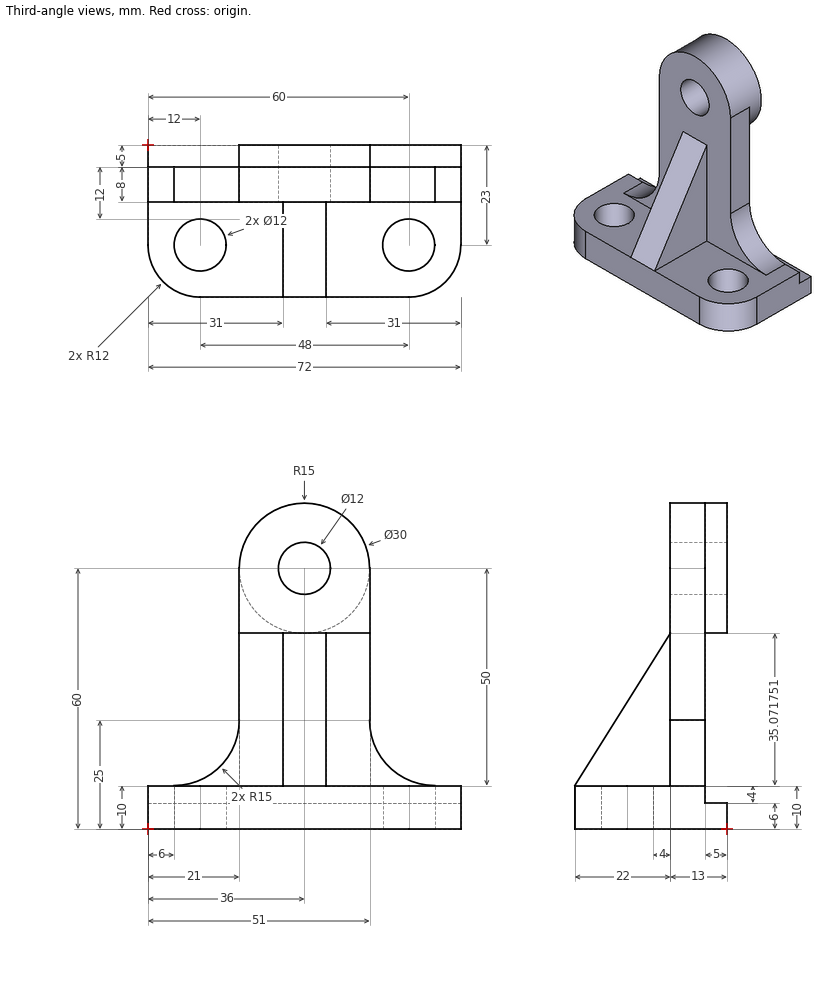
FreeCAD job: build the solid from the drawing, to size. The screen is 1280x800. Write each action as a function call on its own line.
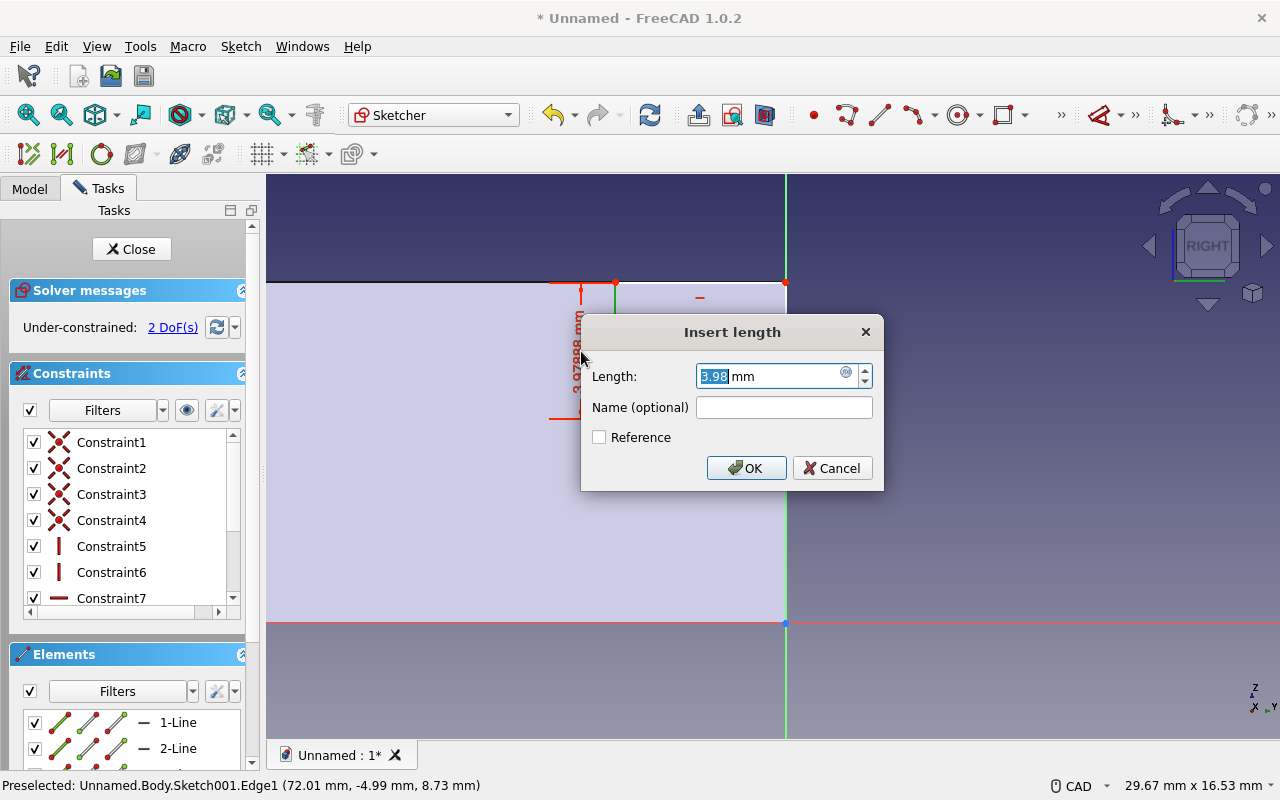
text(4)
key(Return)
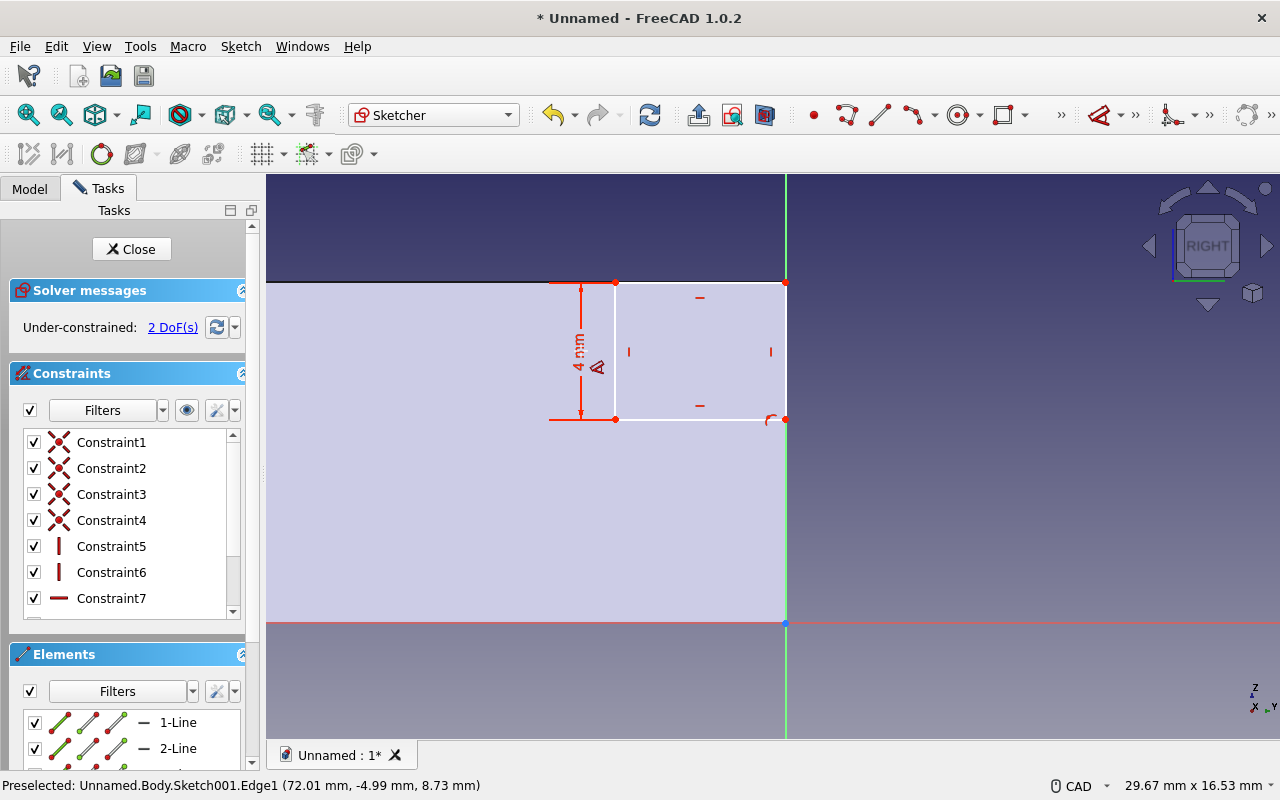
click(666, 420)
click(700, 386)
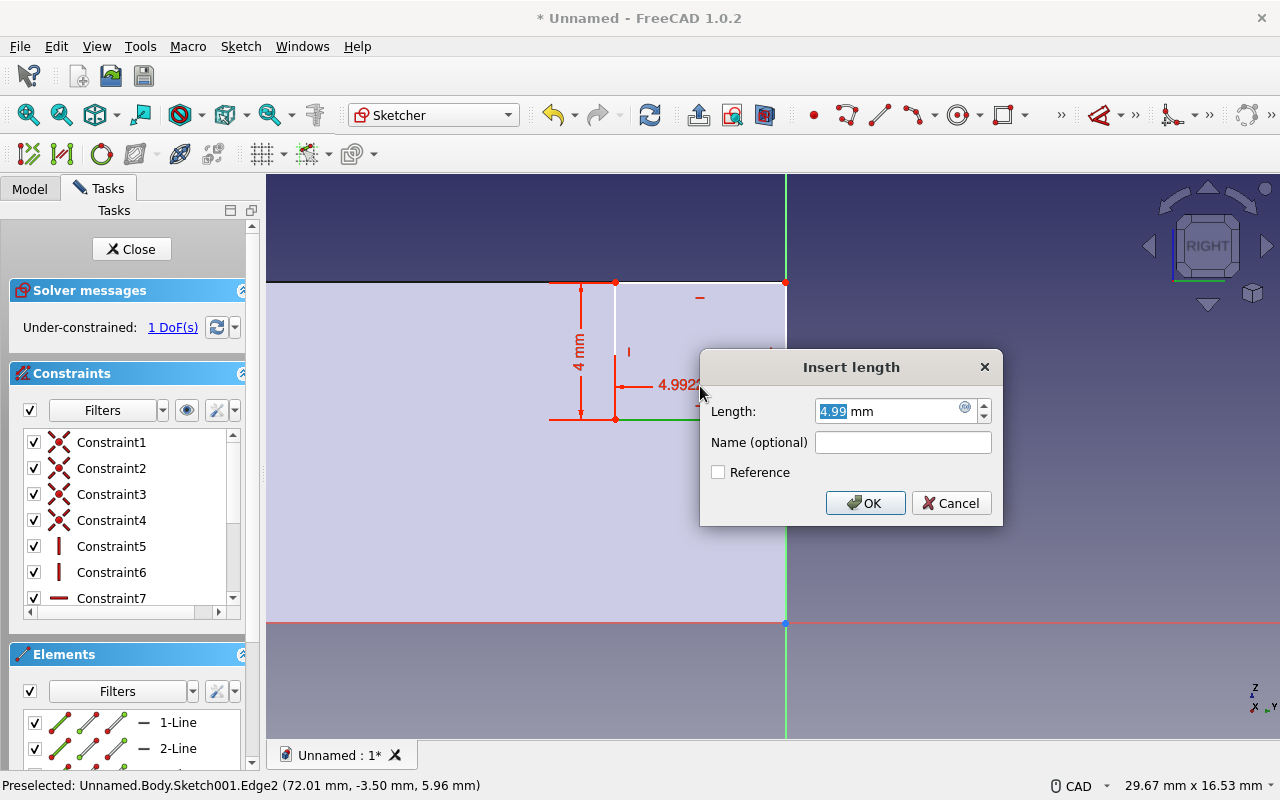
text(5)
key(Return)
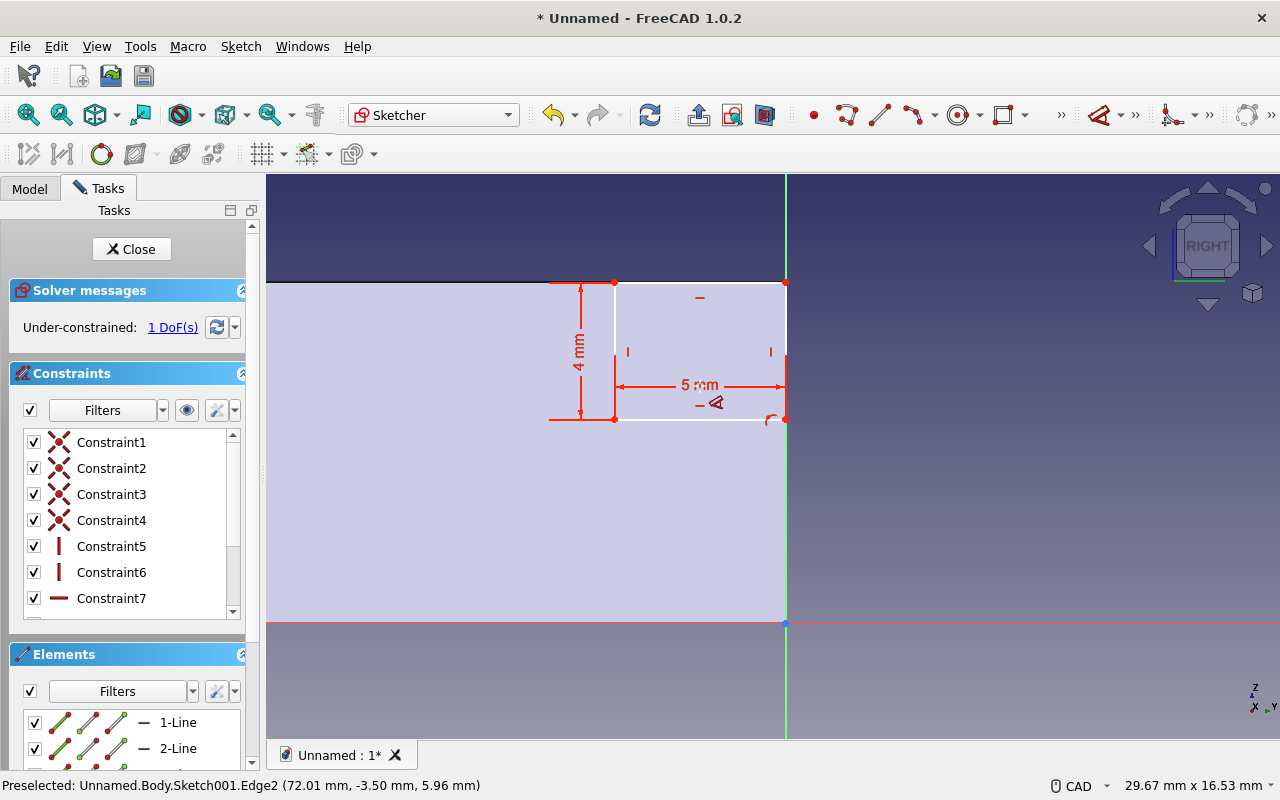
click(615, 420)
click(820, 522)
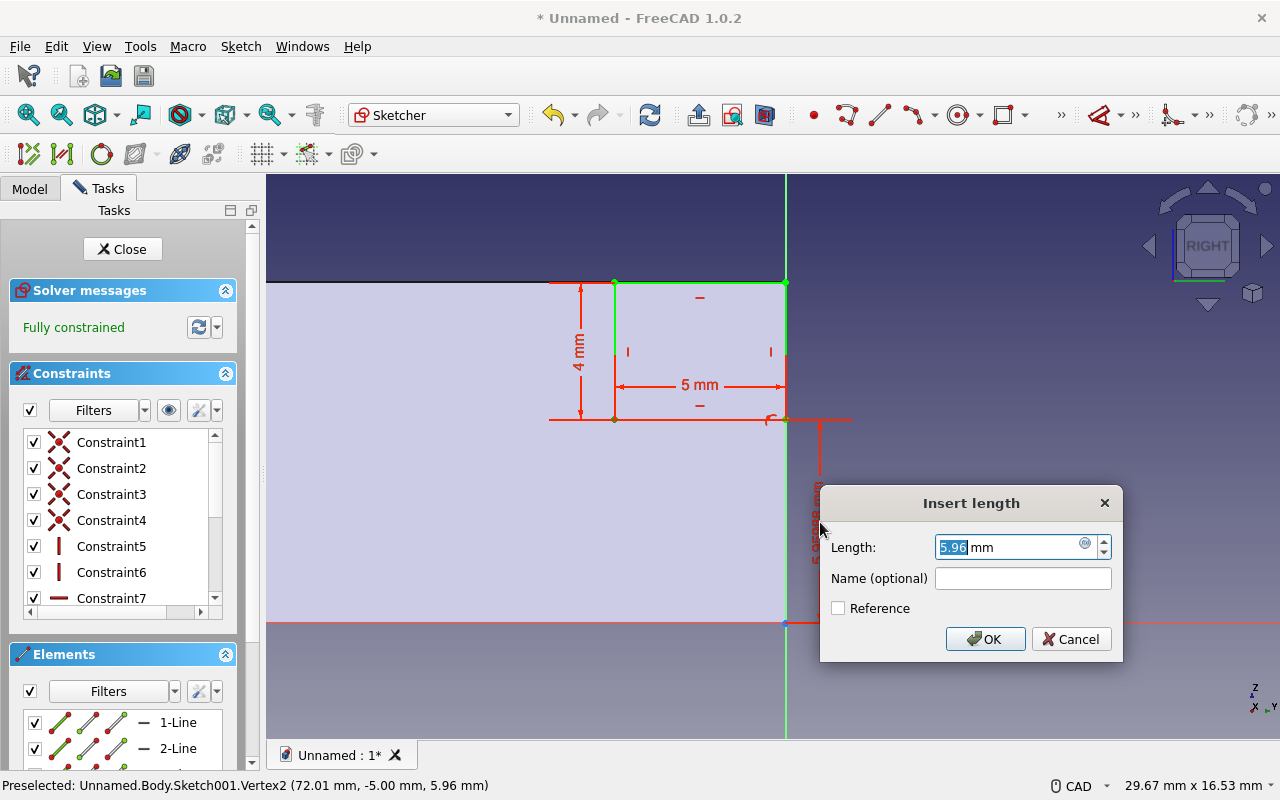
text(6)
key(Return)
key(Escape)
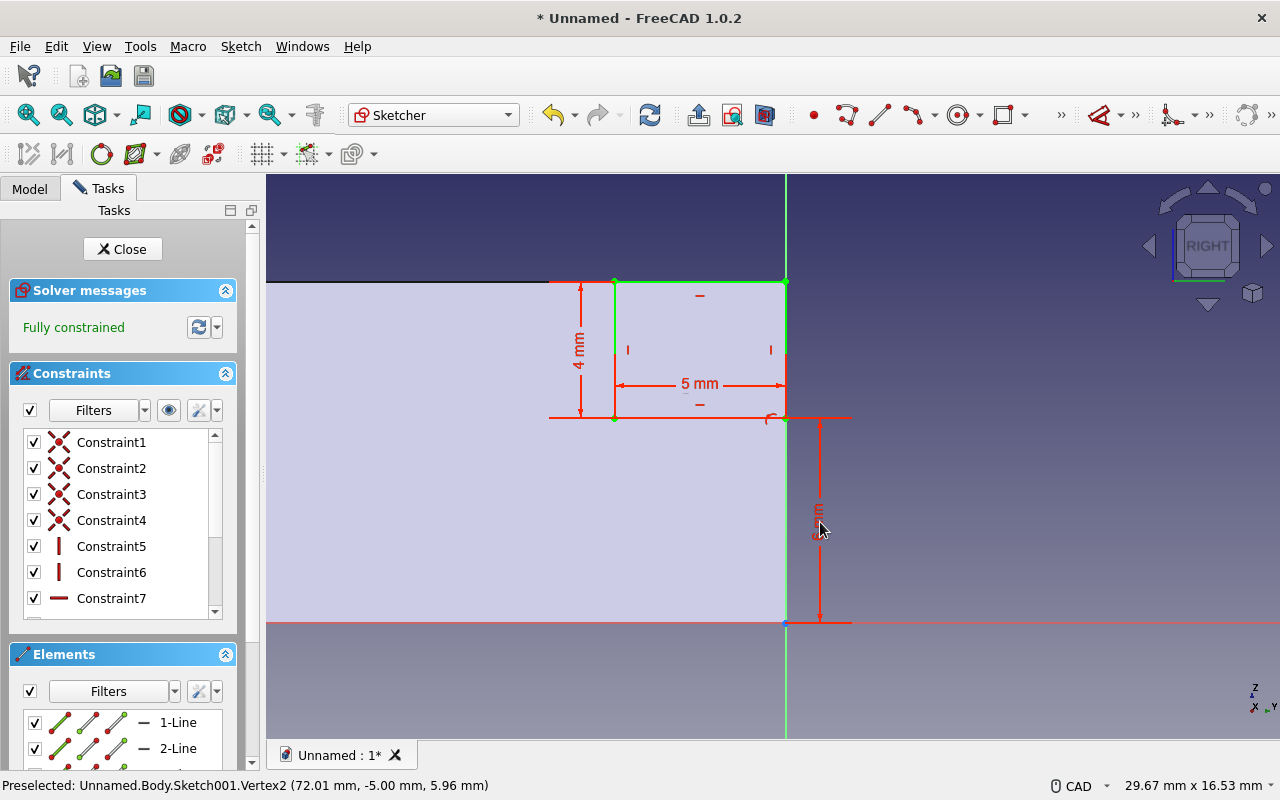
click(123, 249)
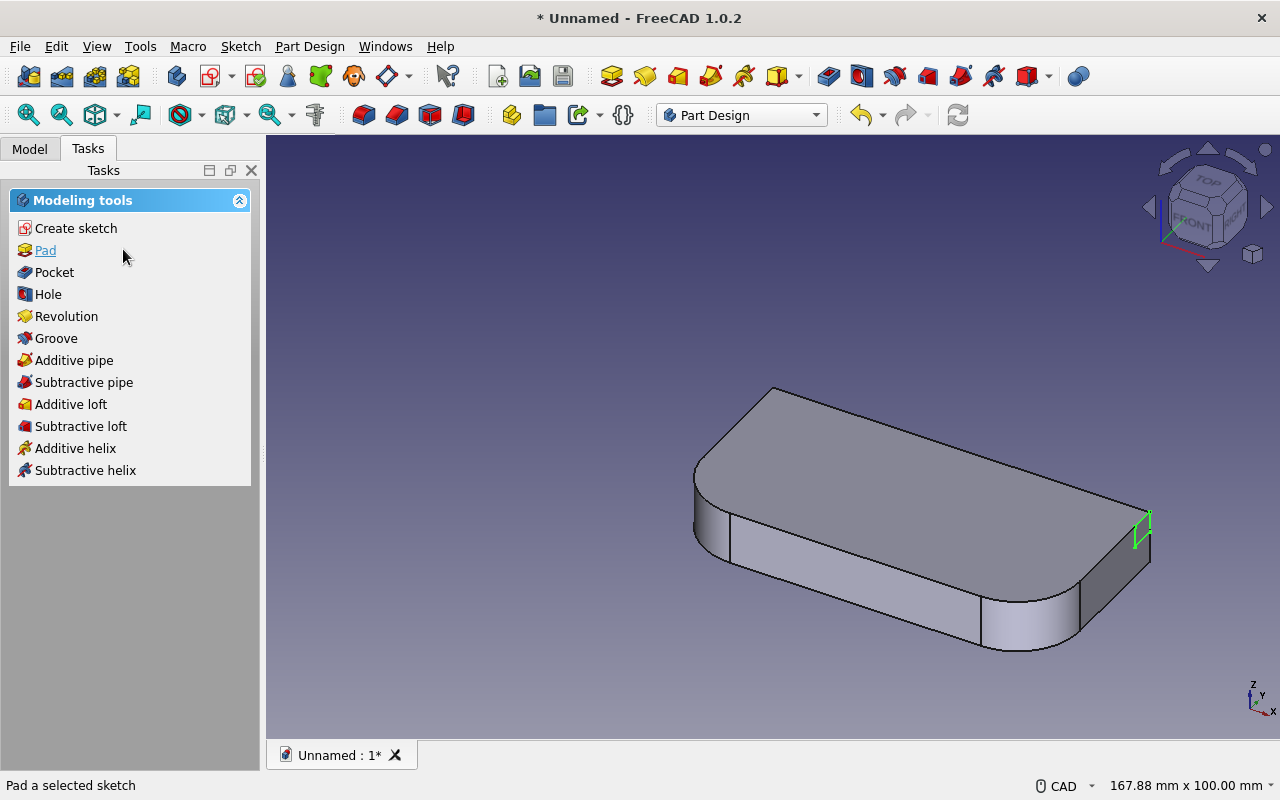
click(829, 76)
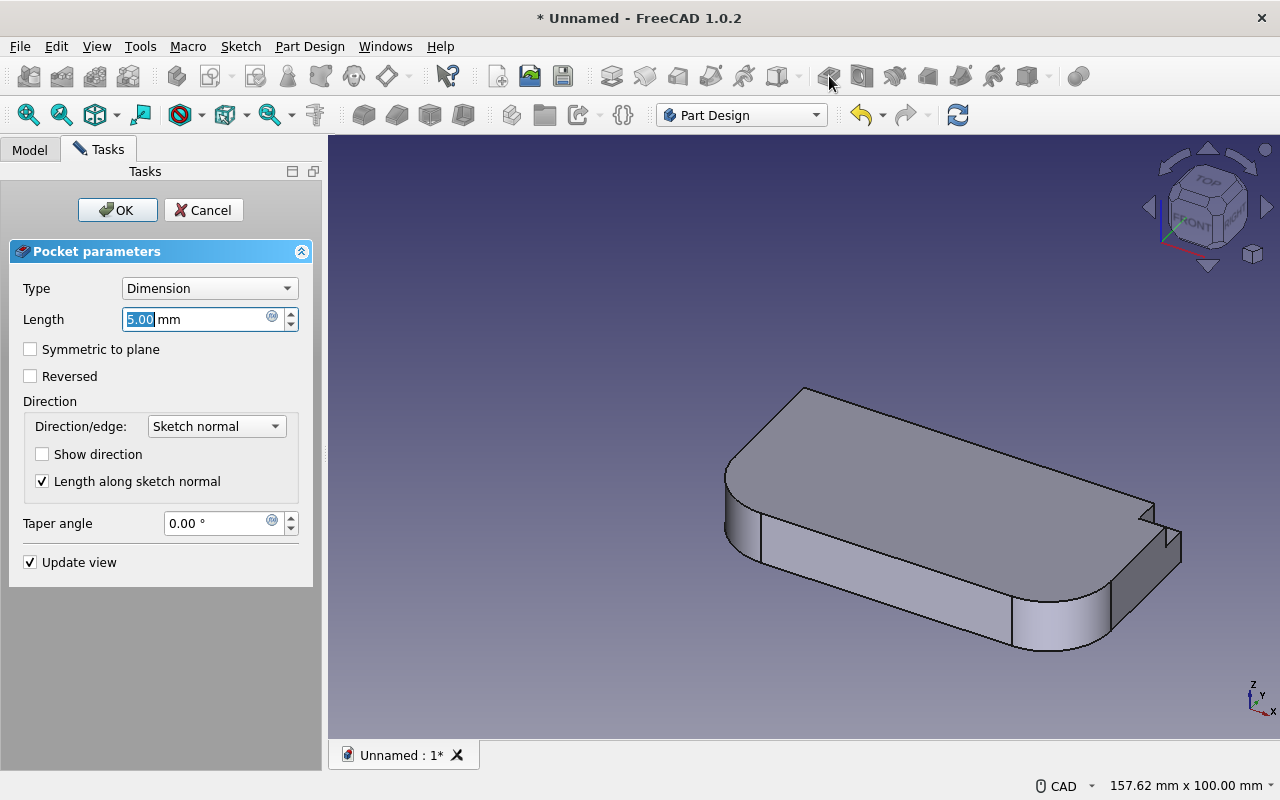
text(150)
key(Tab)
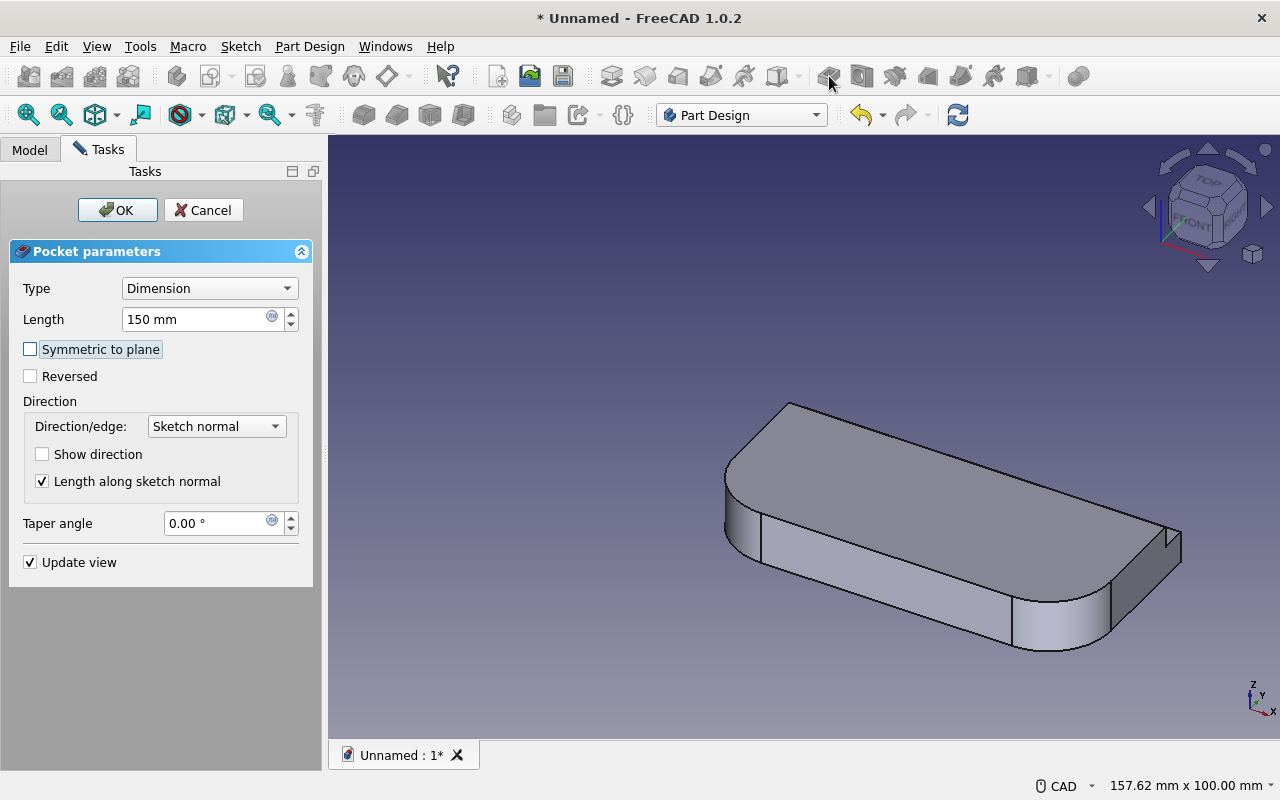
click(118, 210)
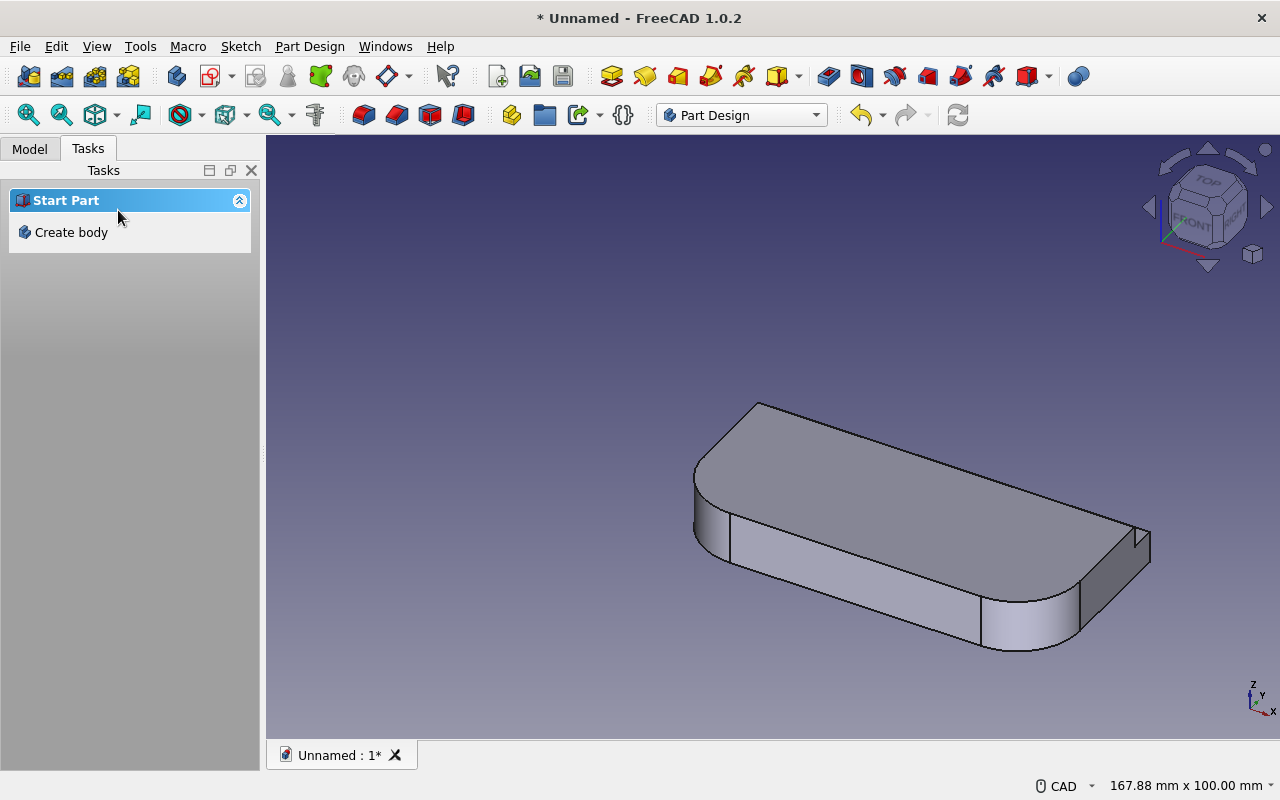
key(4)